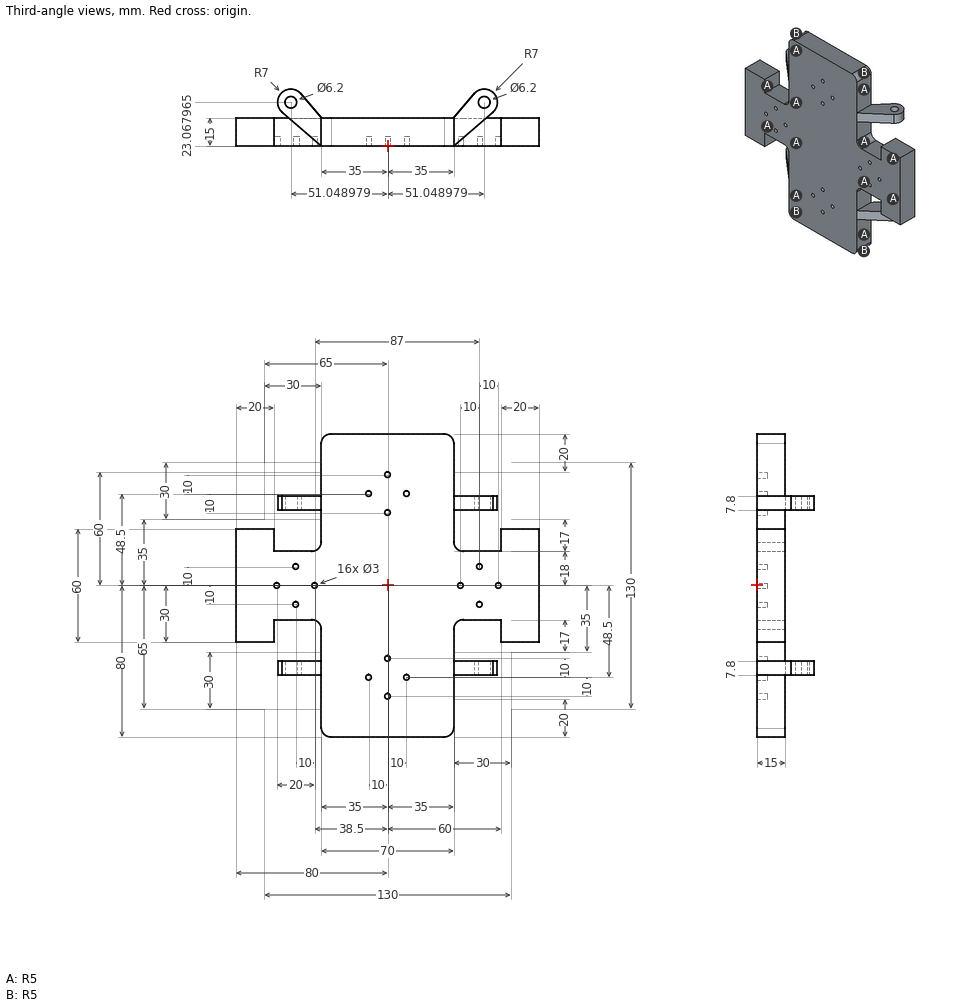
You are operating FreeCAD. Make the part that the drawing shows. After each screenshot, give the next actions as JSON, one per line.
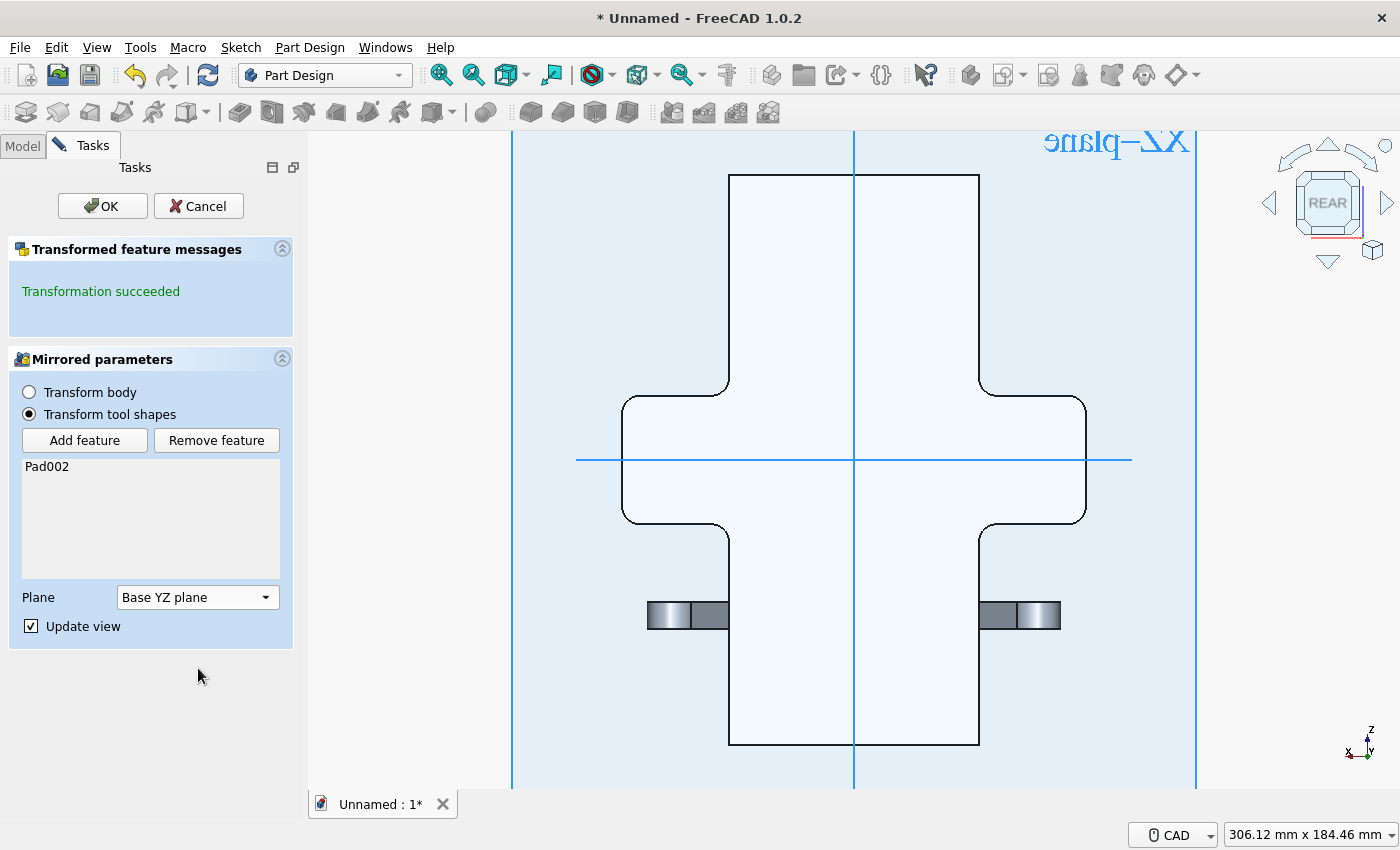
{"action": "left_click", "coordinate": [103, 206]}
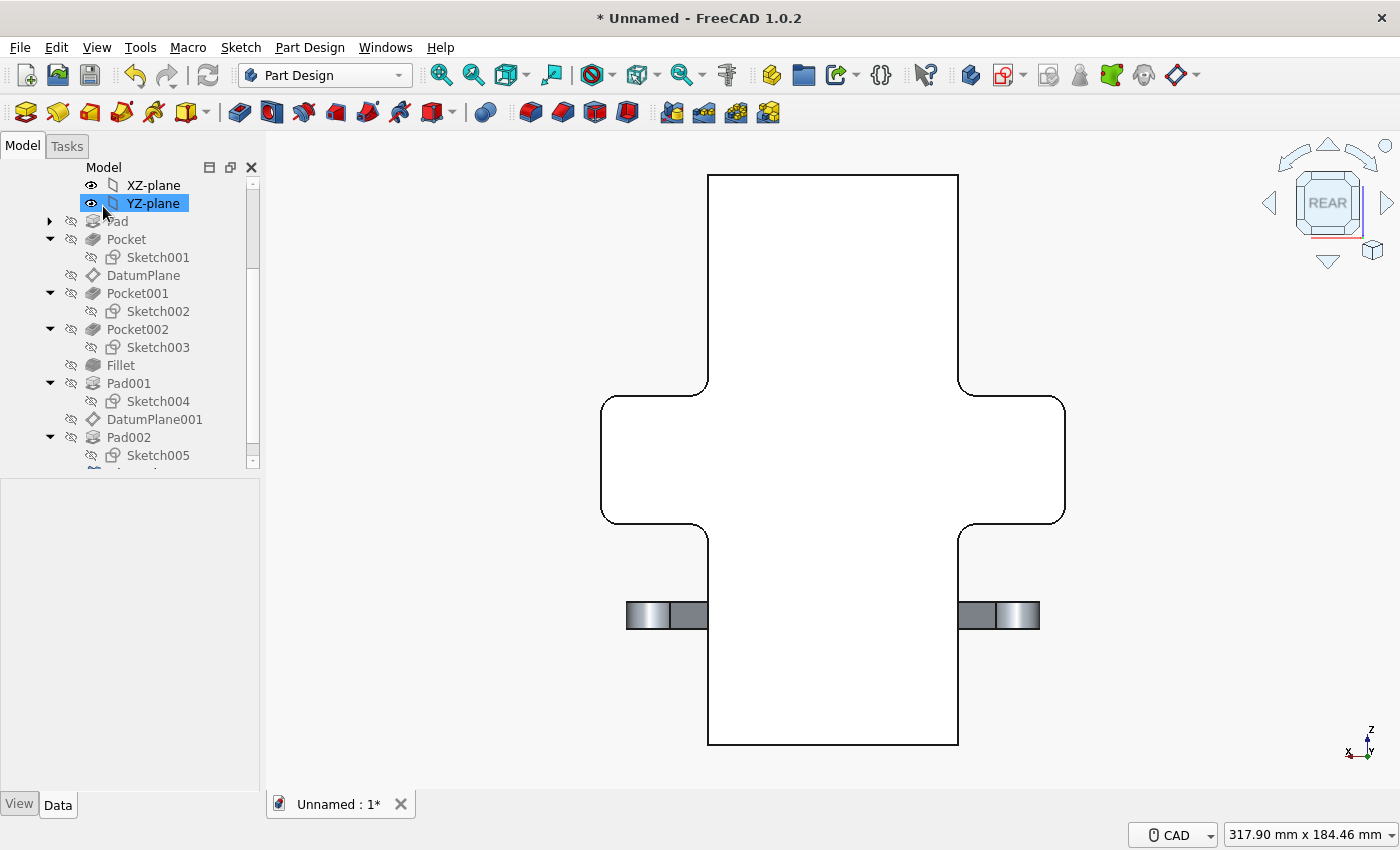
{"action": "left_click", "coordinate": [116, 437]}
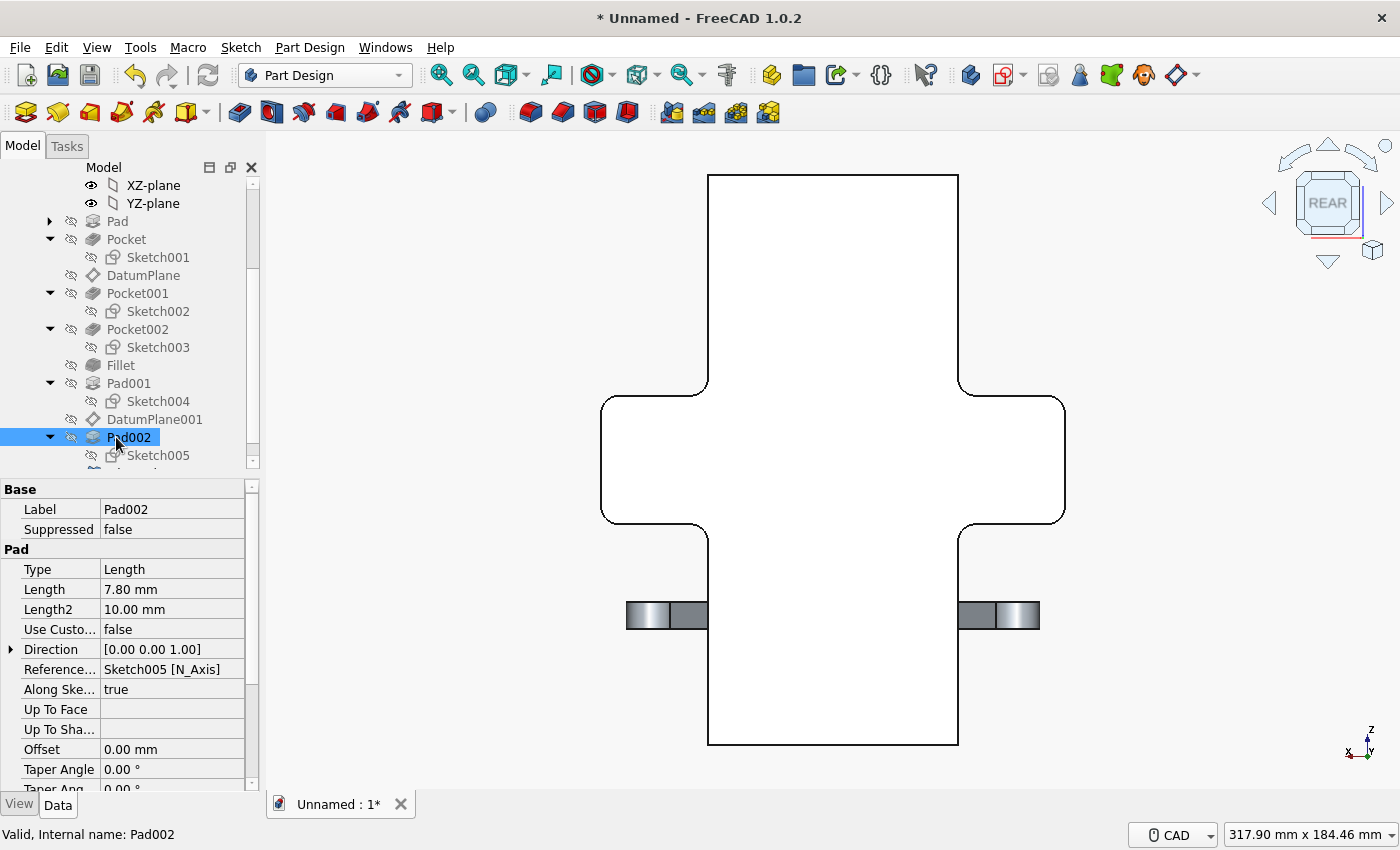
{"action": "left_click", "coordinate": [672, 112]}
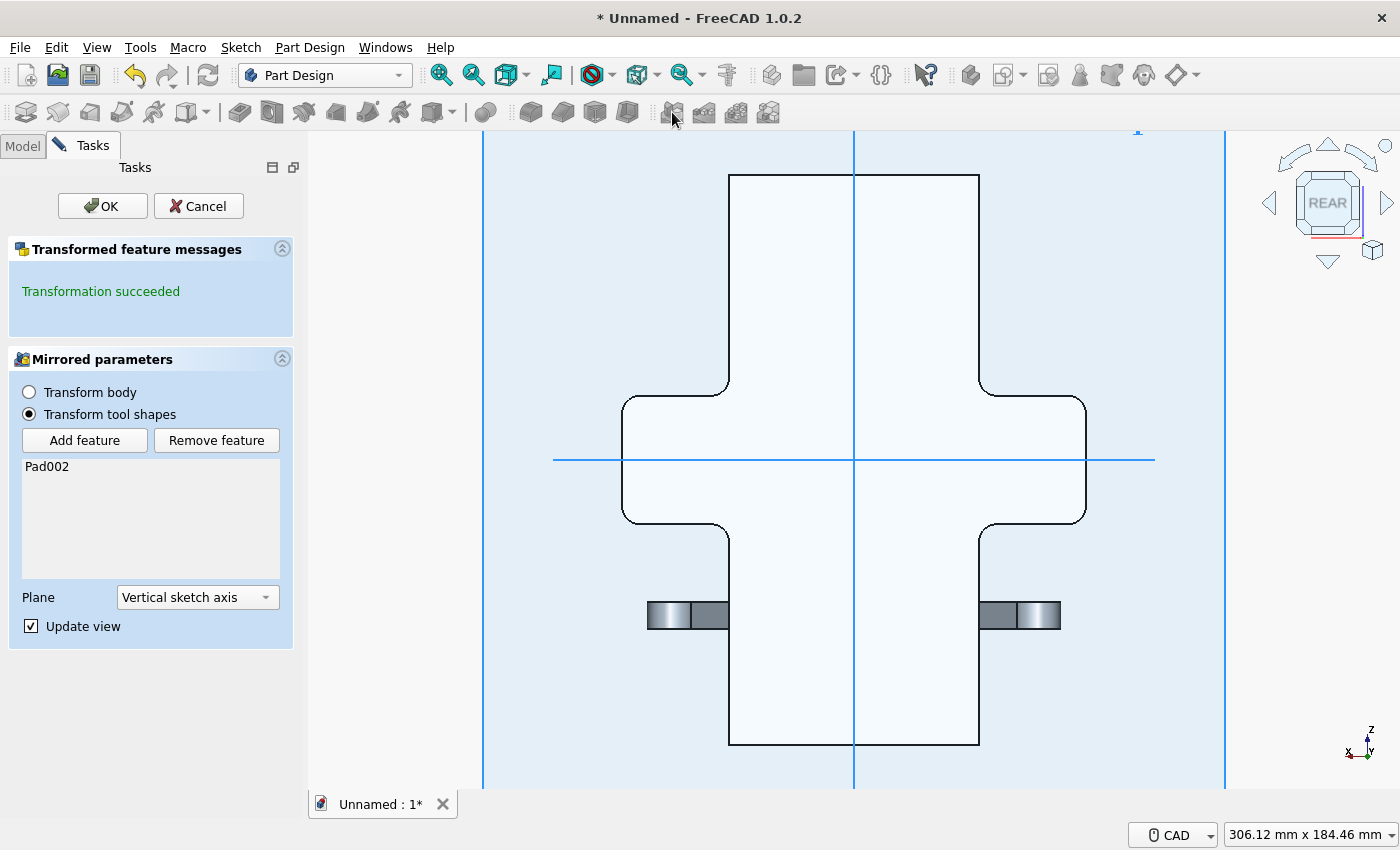
{"action": "left_click", "coordinate": [198, 598]}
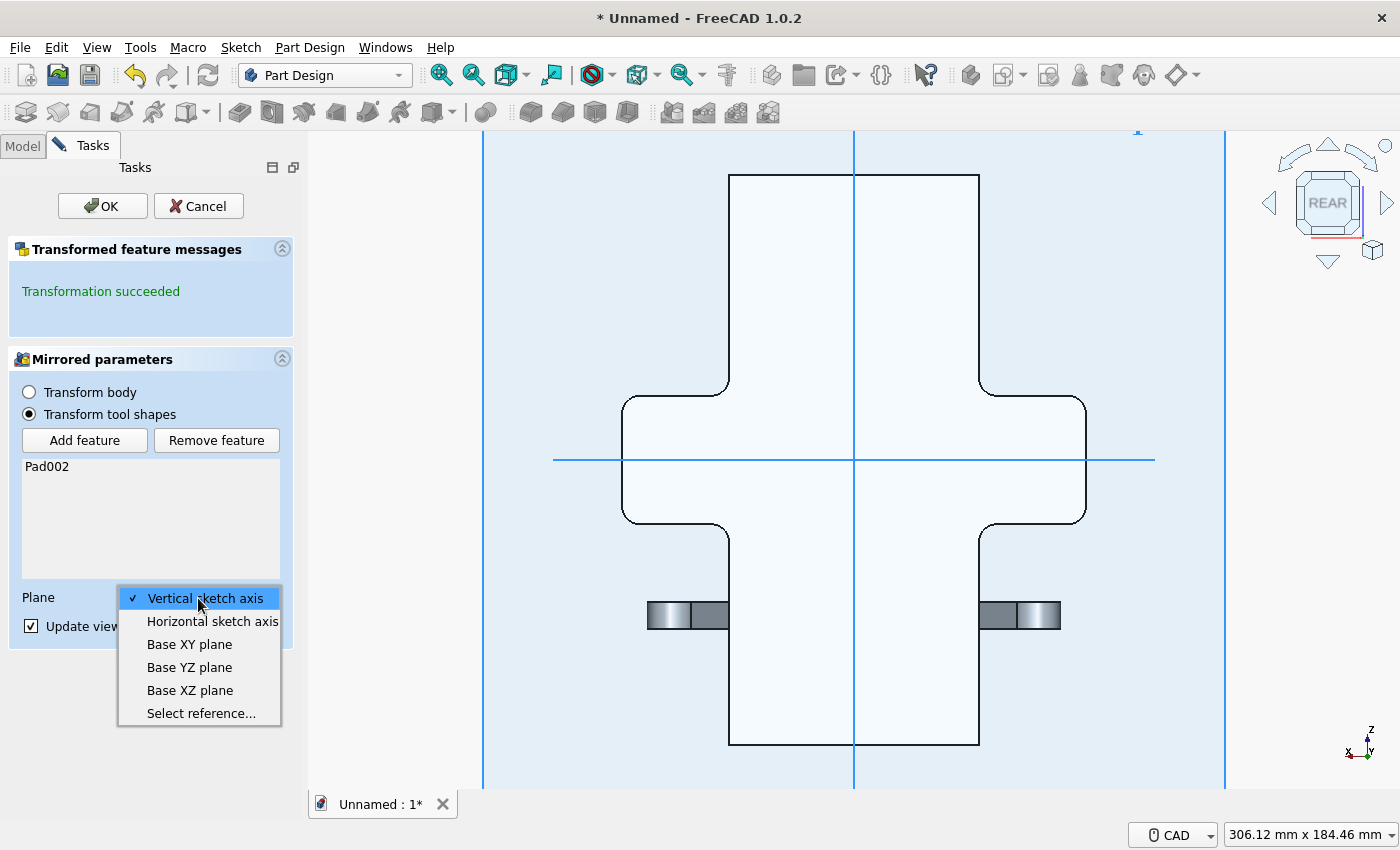
{"action": "left_click", "coordinate": [198, 644]}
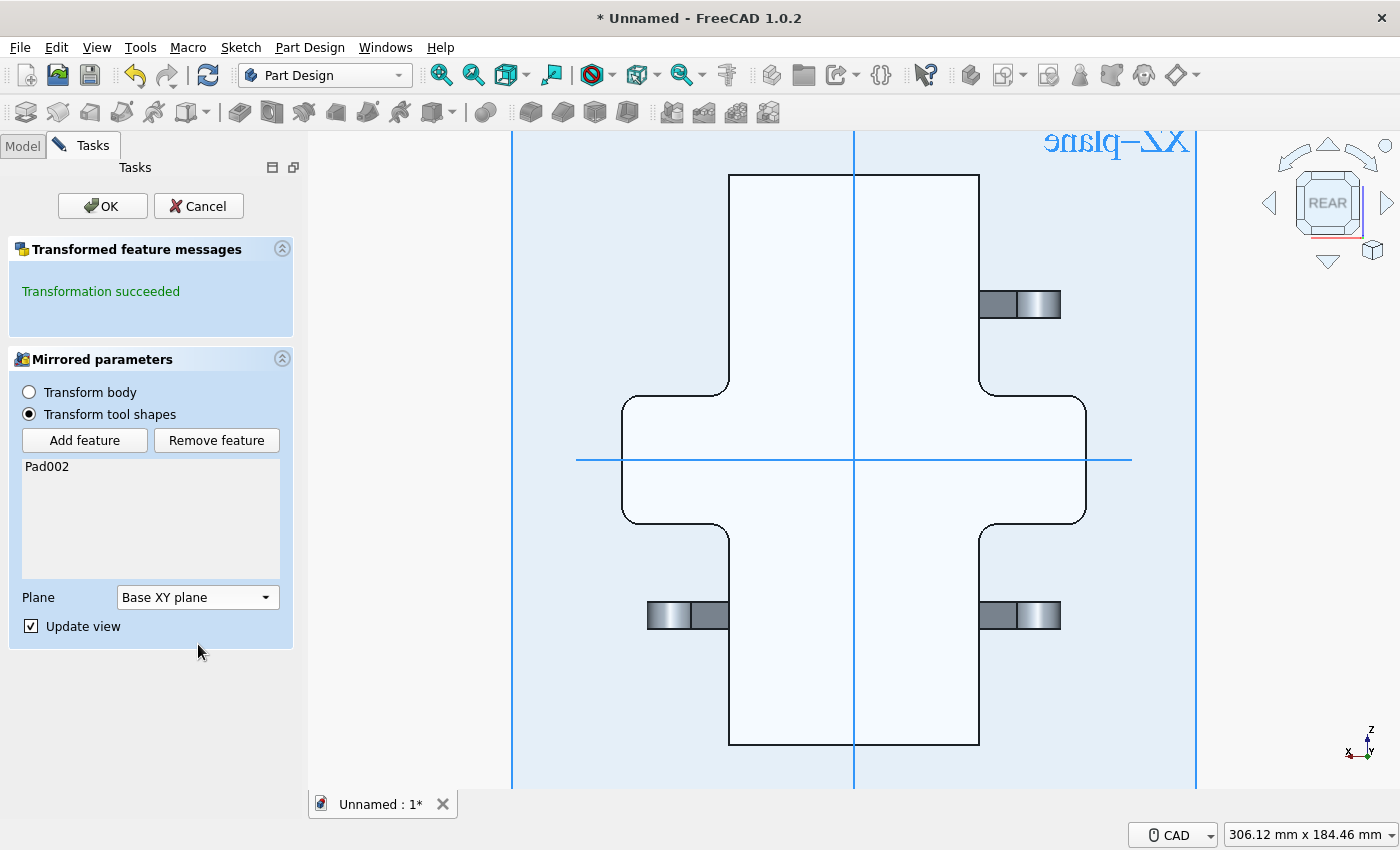
{"action": "left_click", "coordinate": [103, 206]}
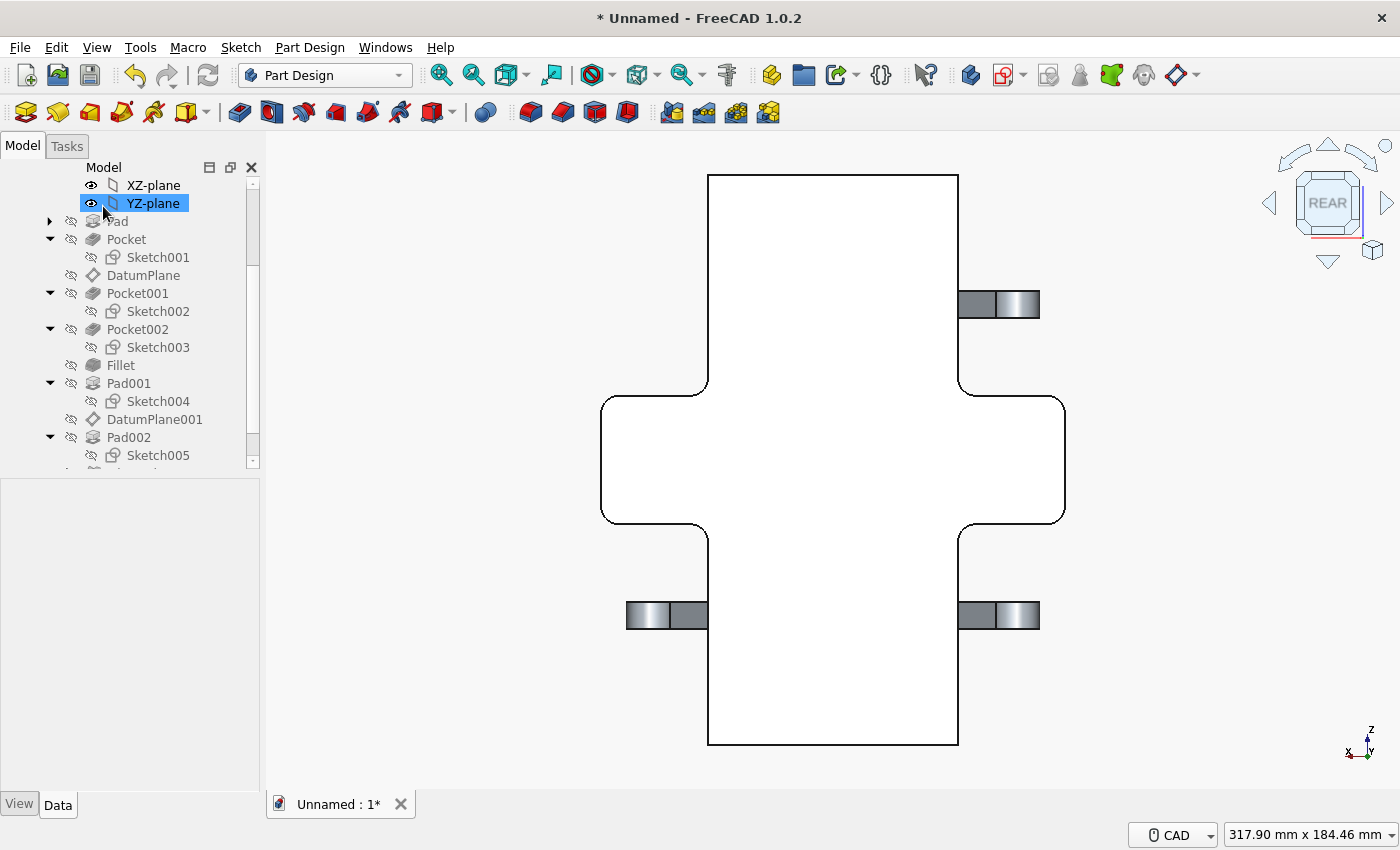
{"action": "scroll", "coordinate": [160, 325], "scroll_direction": "down", "scroll_amount": 3}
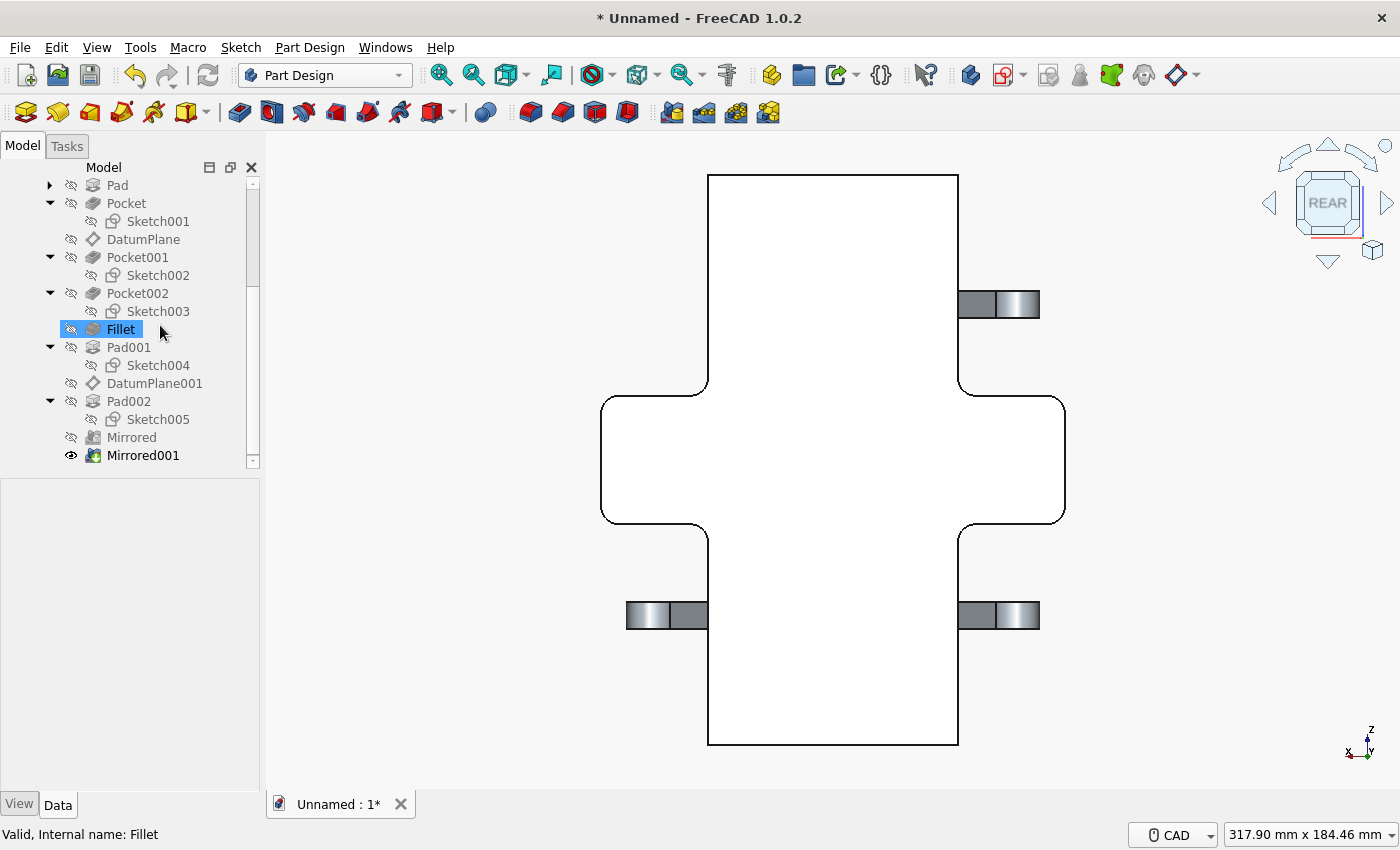
{"action": "scroll", "coordinate": [140, 325], "scroll_direction": "up", "scroll_amount": 15}